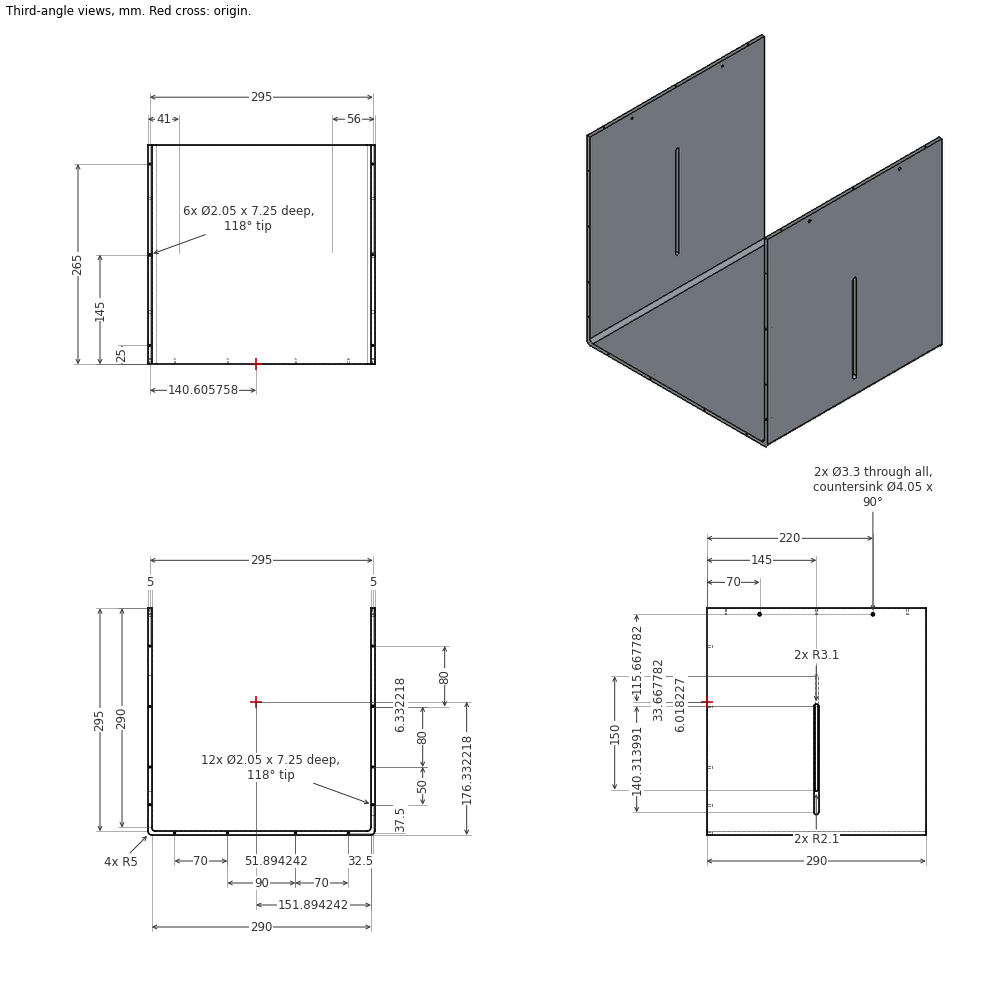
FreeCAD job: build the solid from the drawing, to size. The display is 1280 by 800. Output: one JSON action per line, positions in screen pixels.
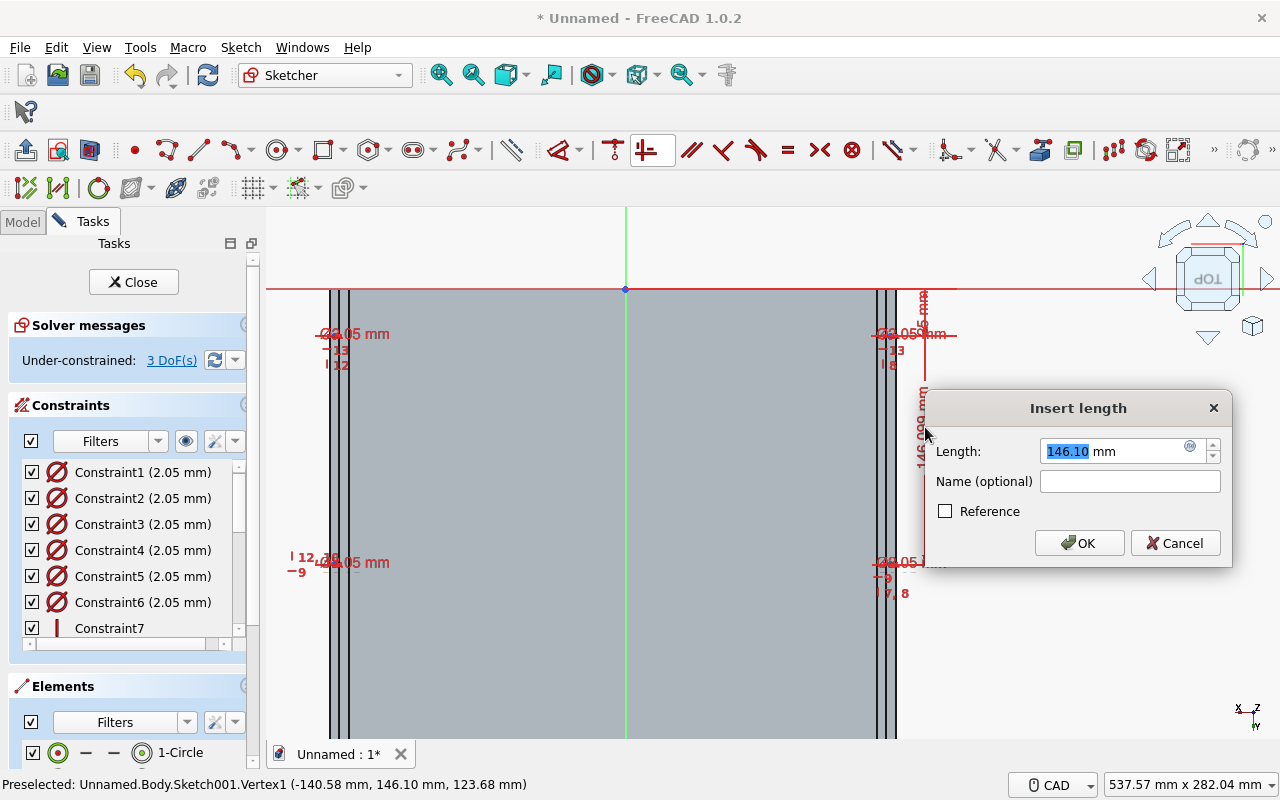
{"action": "type", "text": "145"}
{"action": "key", "text": "Return"}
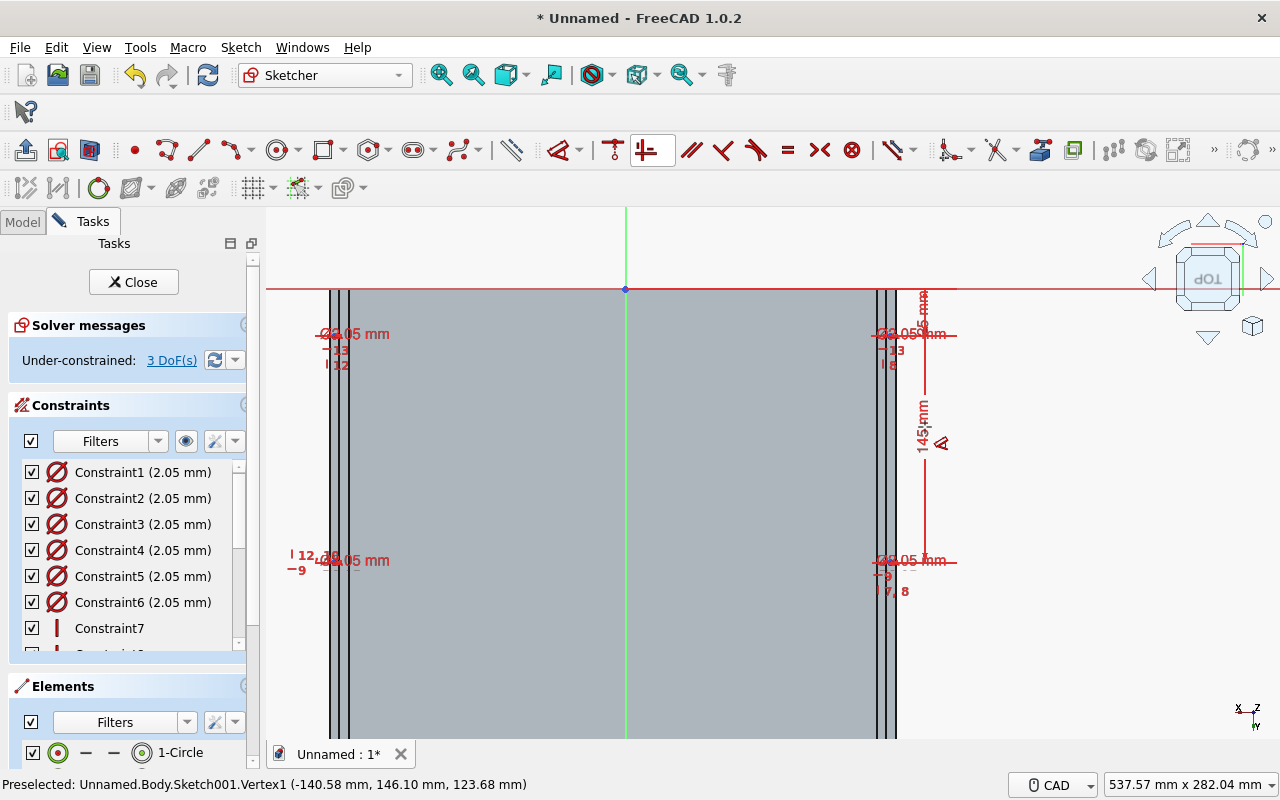
{"action": "scroll", "coordinate": [891, 337], "scroll_direction": "down", "scroll_amount": 2}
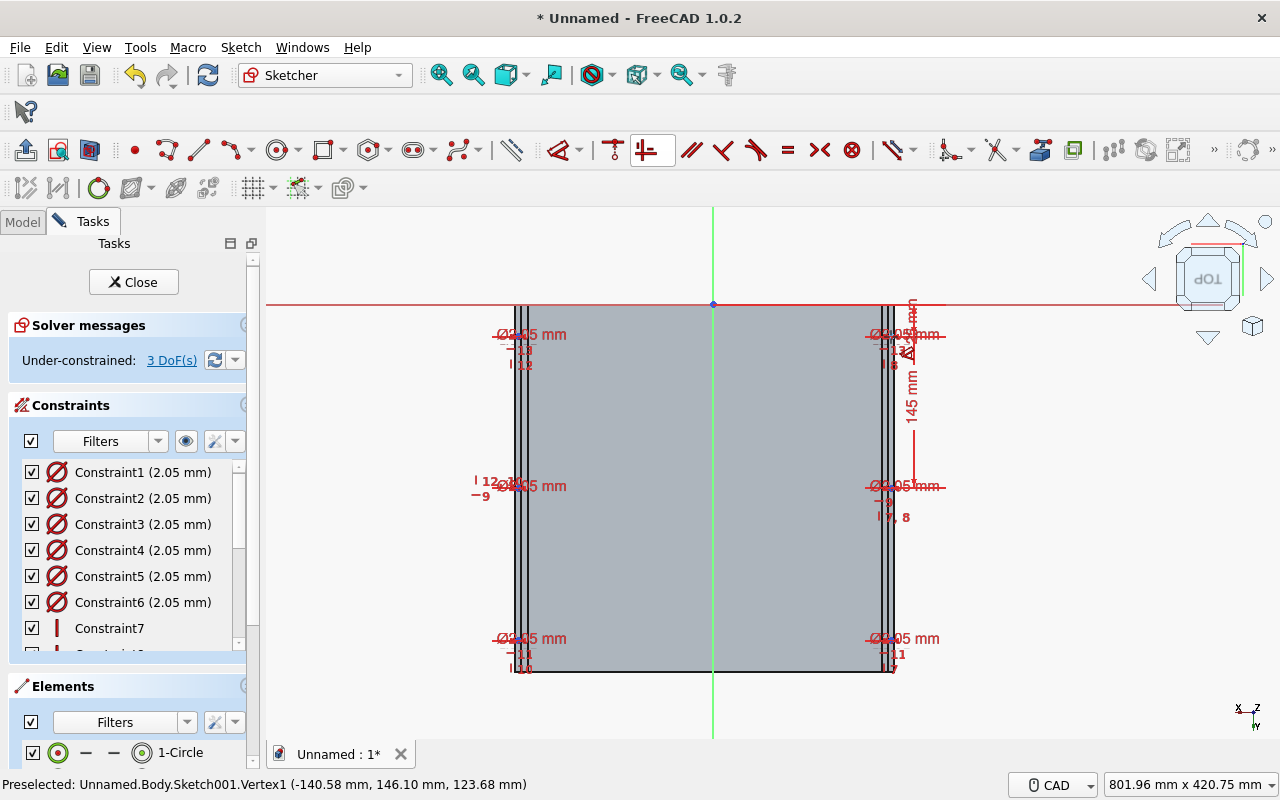
{"action": "left_click", "coordinate": [891, 641]}
{"action": "left_click", "coordinate": [925, 473]}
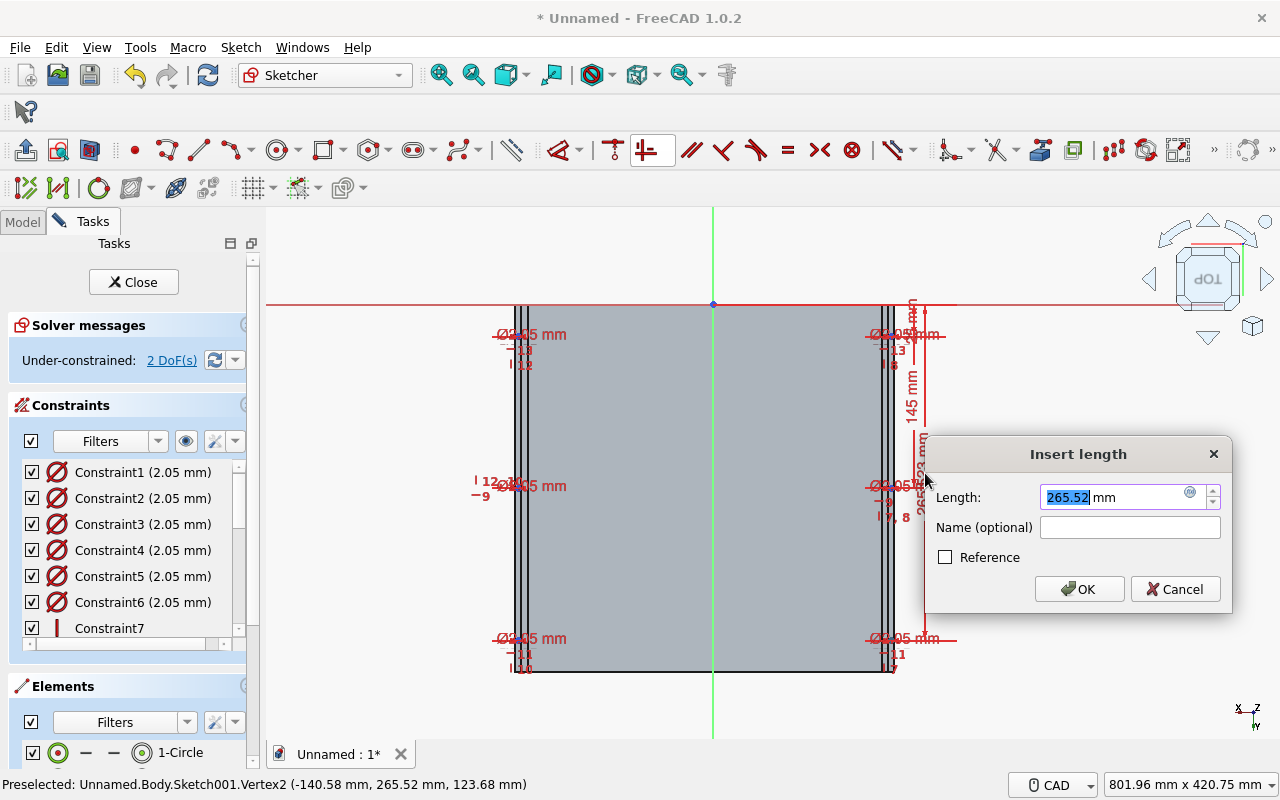
{"action": "type", "text": "265"}
{"action": "key", "text": "Return"}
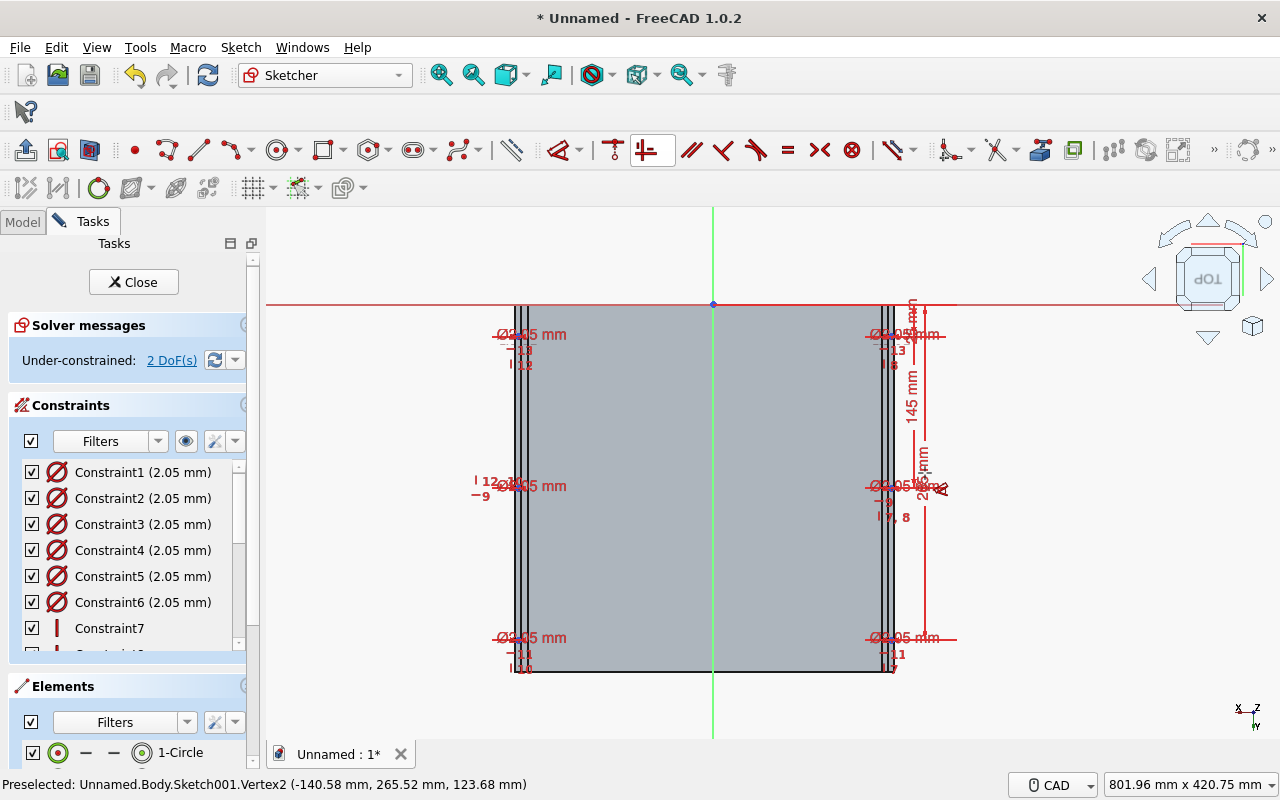
{"action": "left_click", "coordinate": [891, 488]}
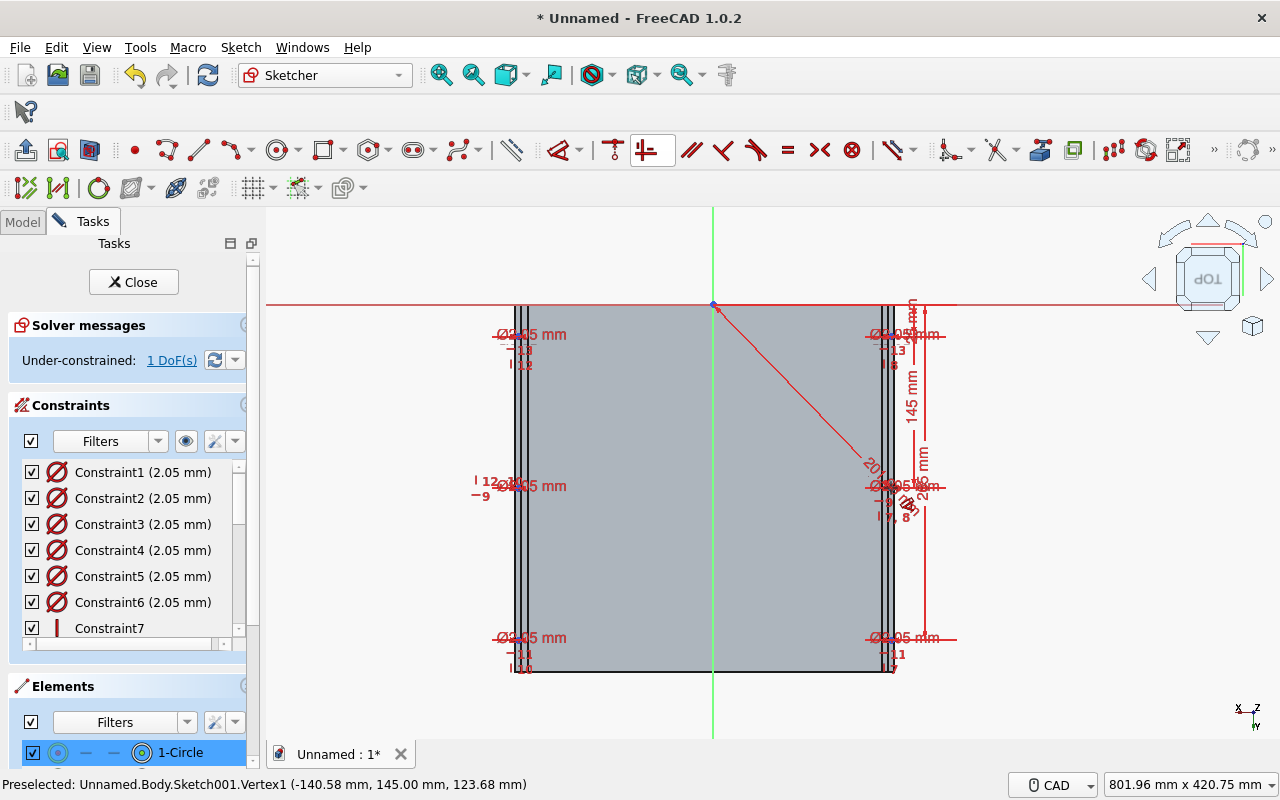
{"action": "left_click", "coordinate": [518, 488]}
{"action": "left_click", "coordinate": [619, 522]}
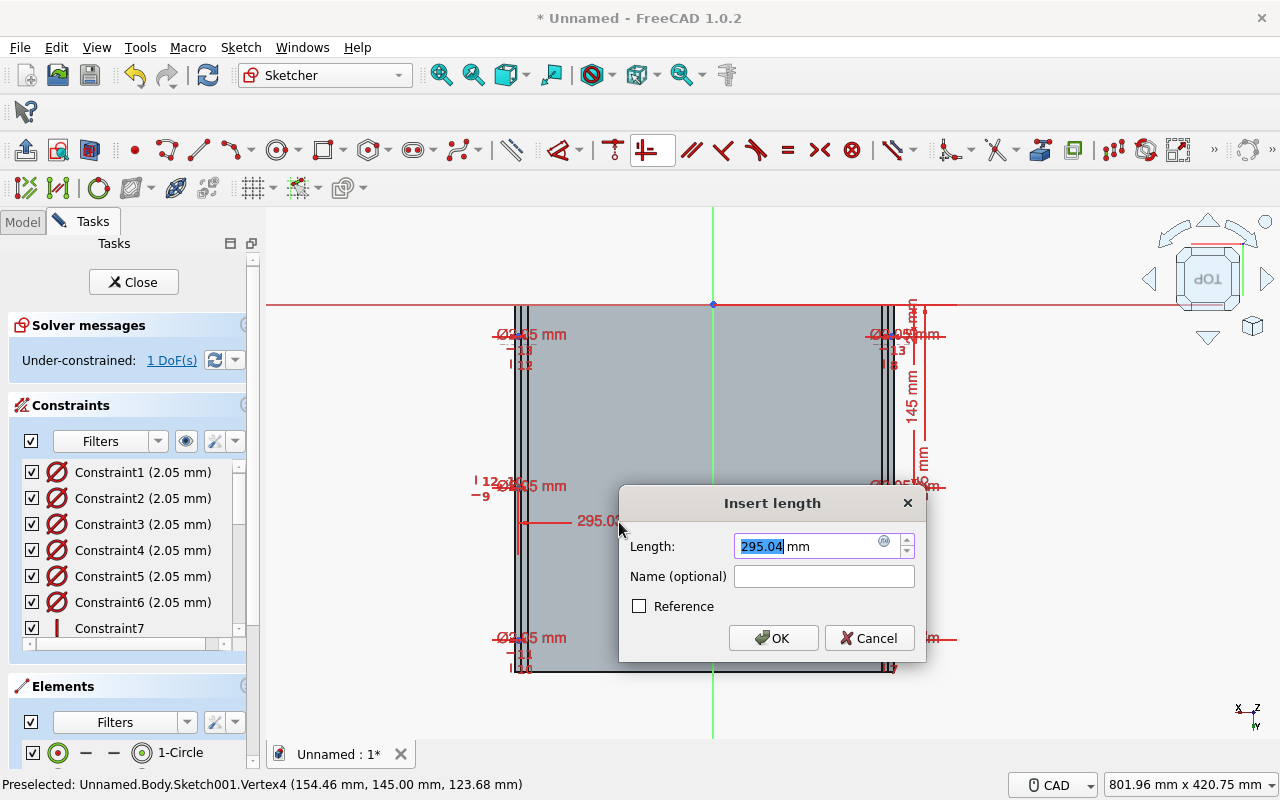
{"action": "type", "text": "295"}
{"action": "key", "text": "Return"}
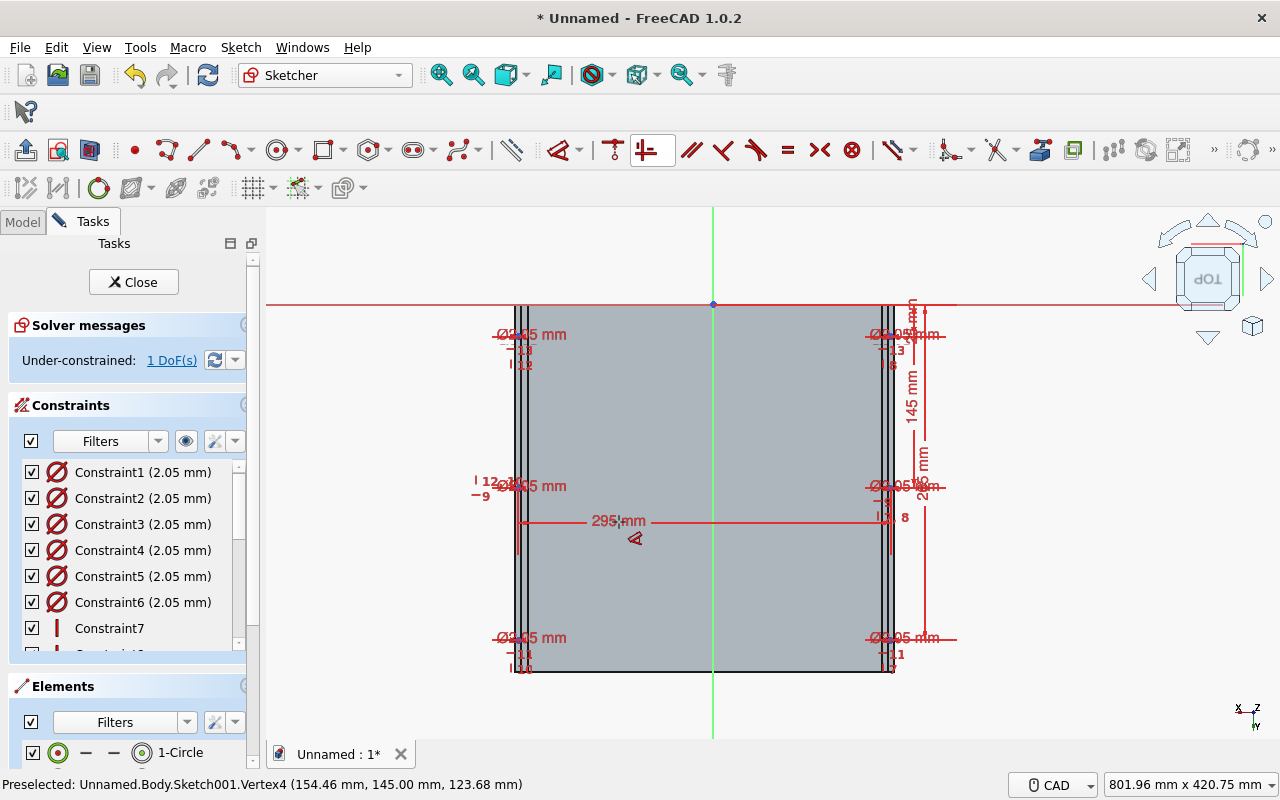
{"action": "left_click", "coordinate": [891, 488]}
{"action": "left_click", "coordinate": [802, 271]}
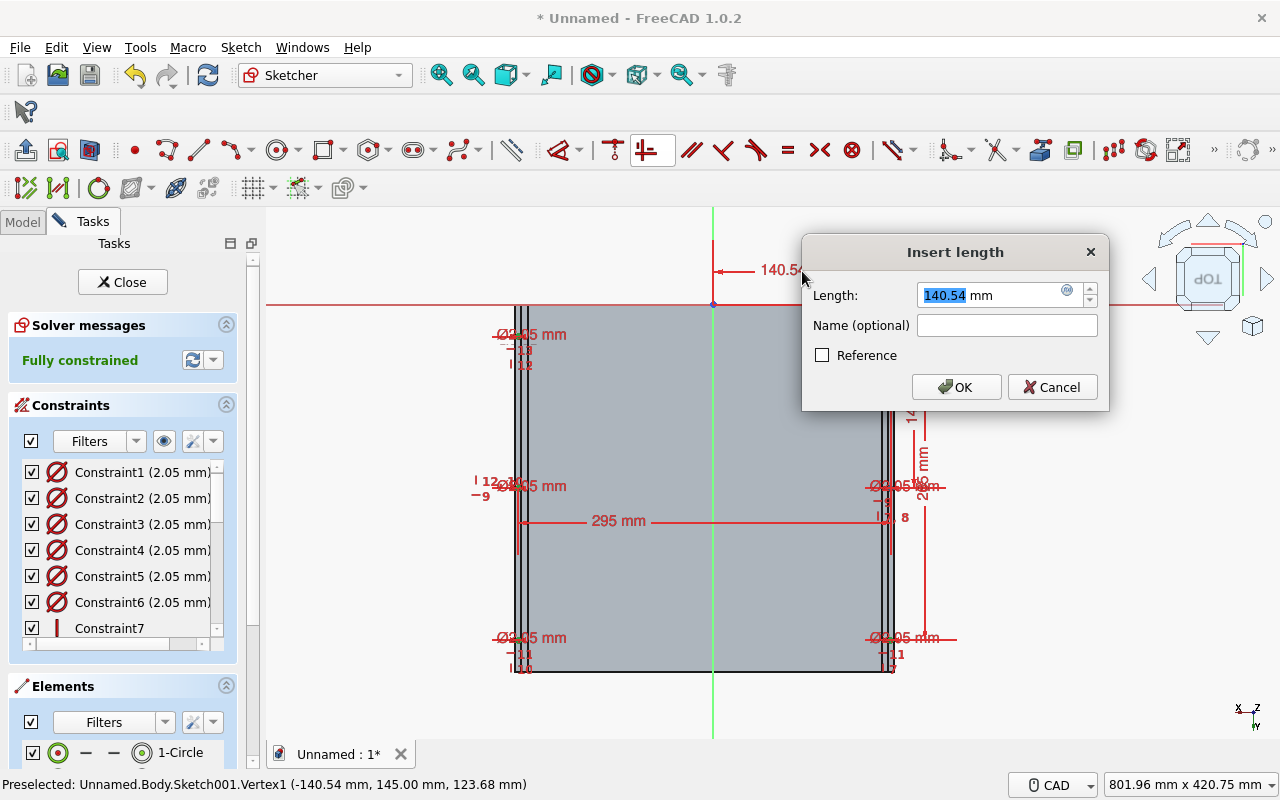
{"action": "type", "text": "140.605758"}
{"action": "key", "text": "Return"}
{"action": "key", "text": "Escape"}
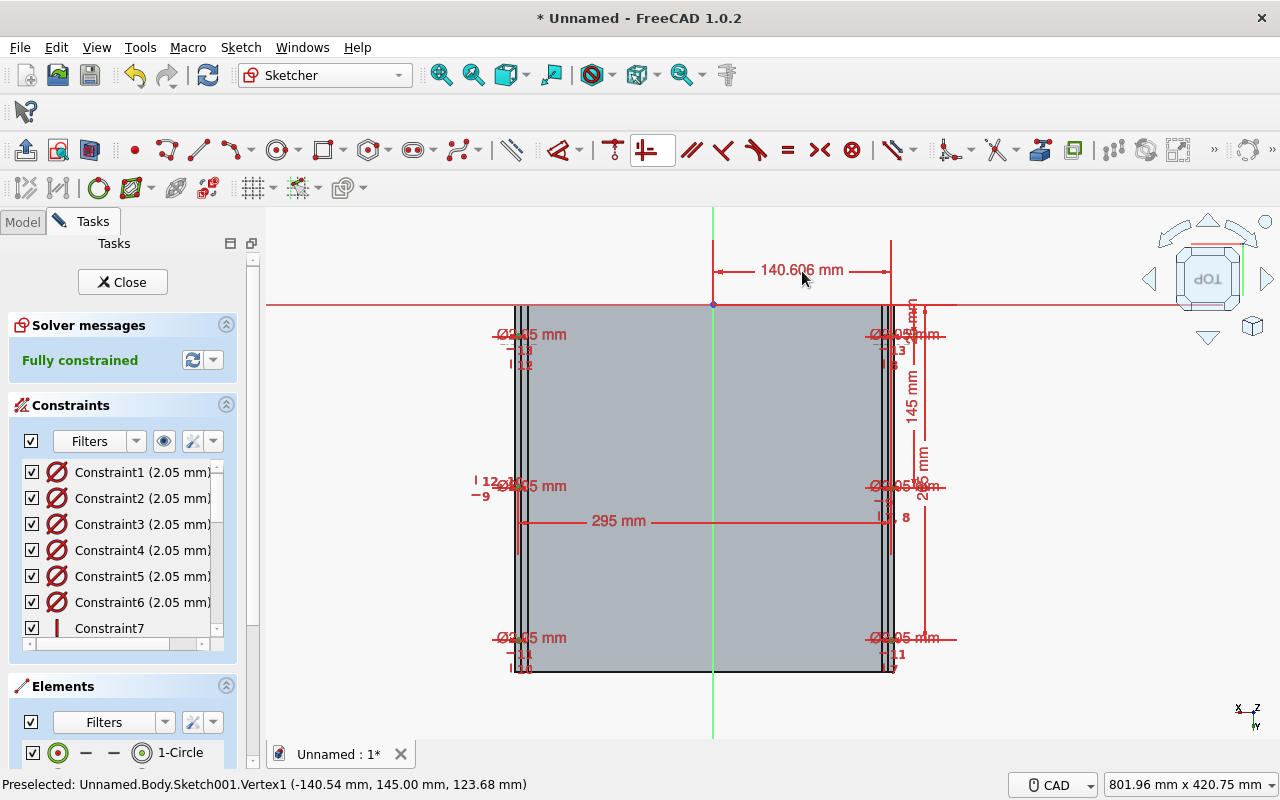
{"action": "left_click", "coordinate": [123, 282]}